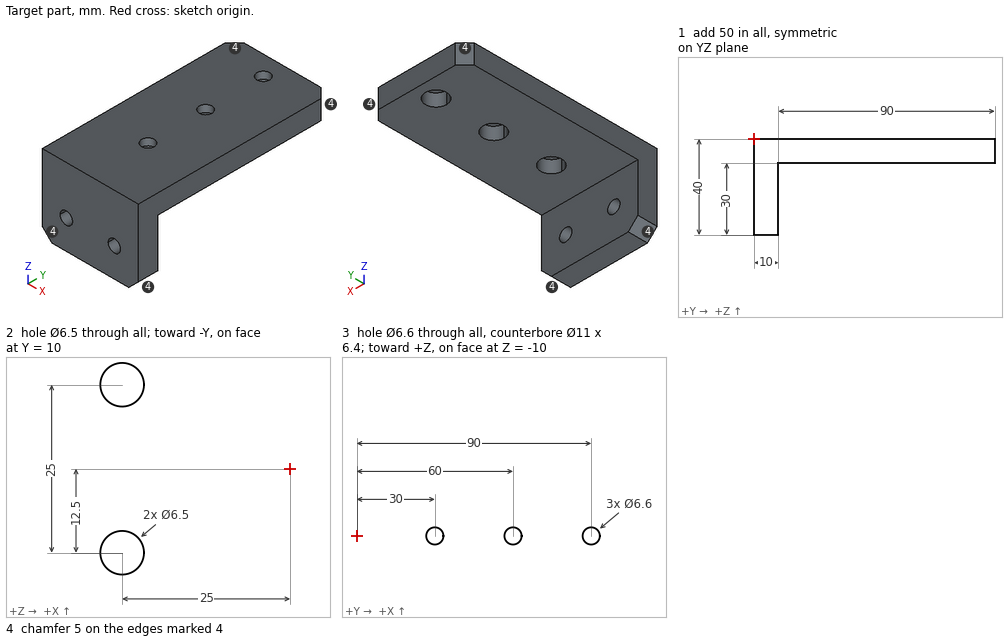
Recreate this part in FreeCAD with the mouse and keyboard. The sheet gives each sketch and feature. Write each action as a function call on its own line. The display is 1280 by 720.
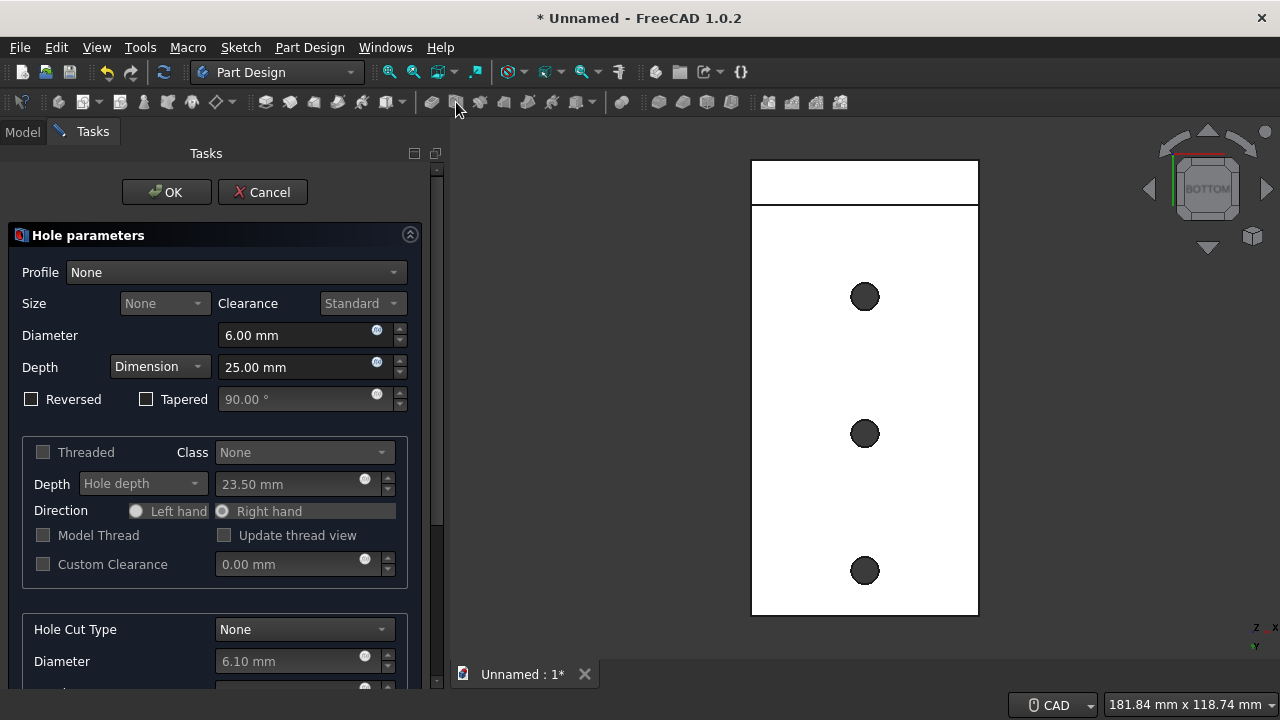
triple_click(305, 335)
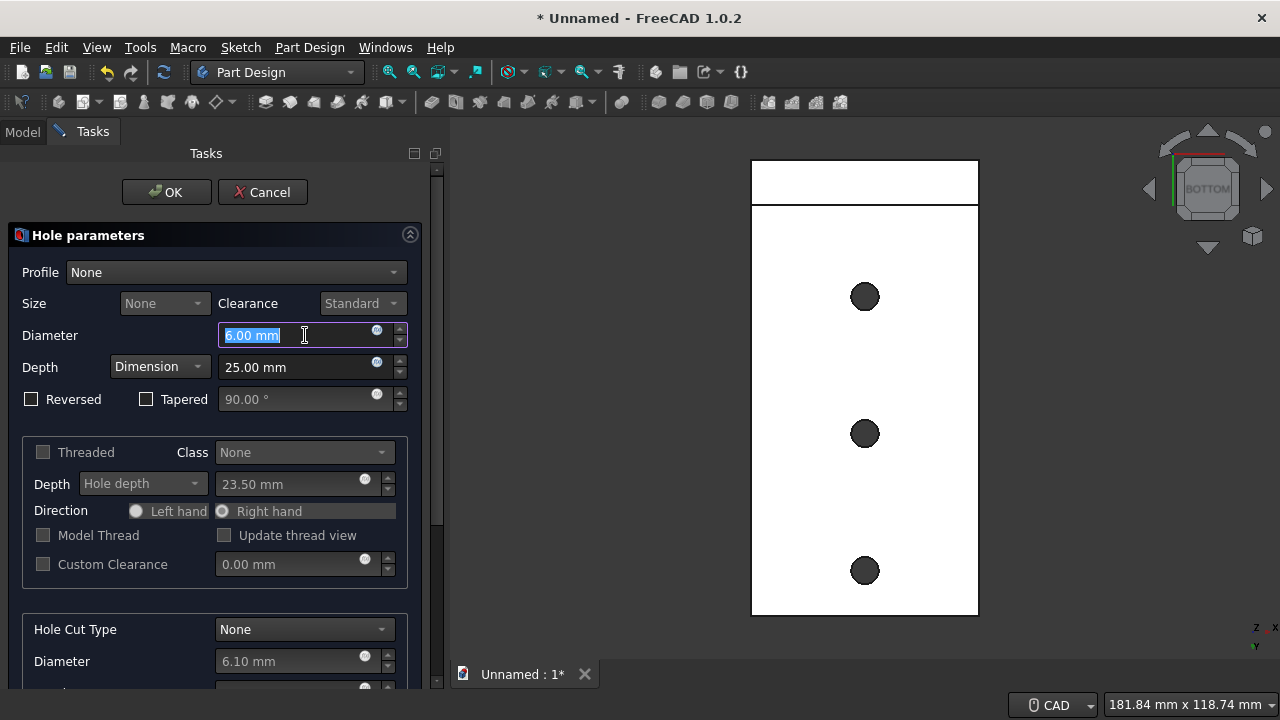
text(6.6)
key(Tab)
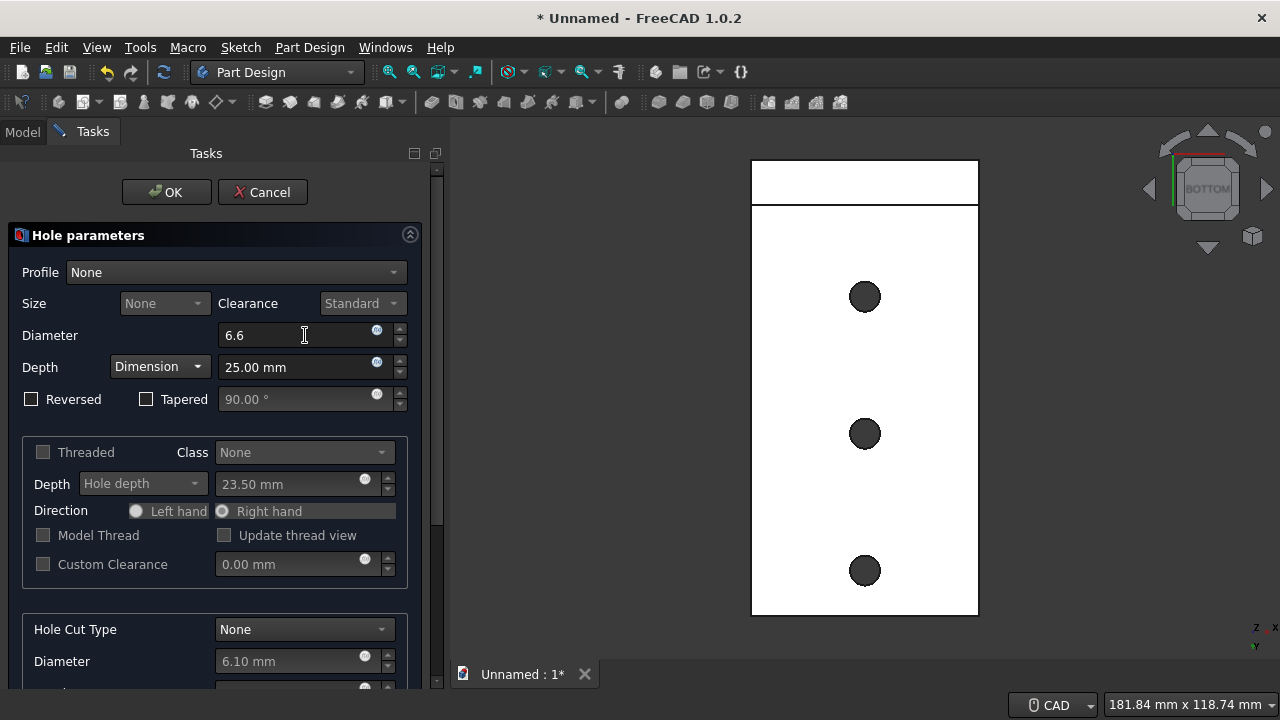
click(161, 366)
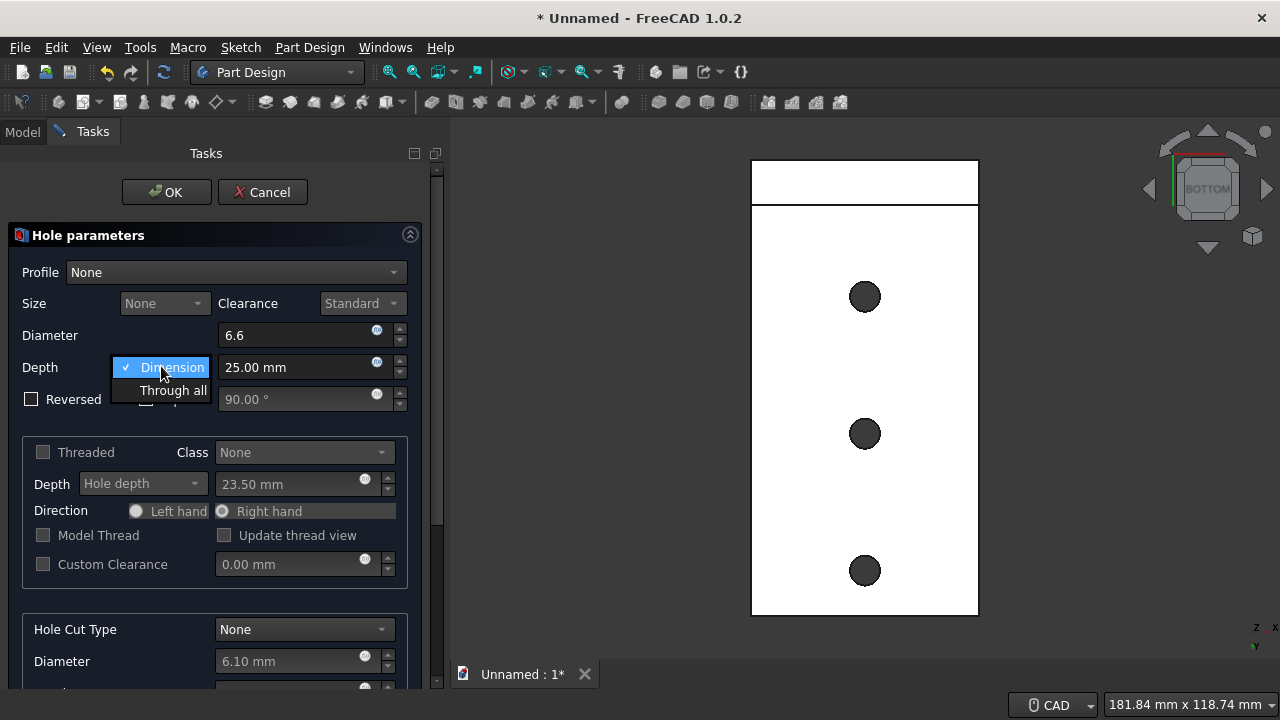
click(160, 390)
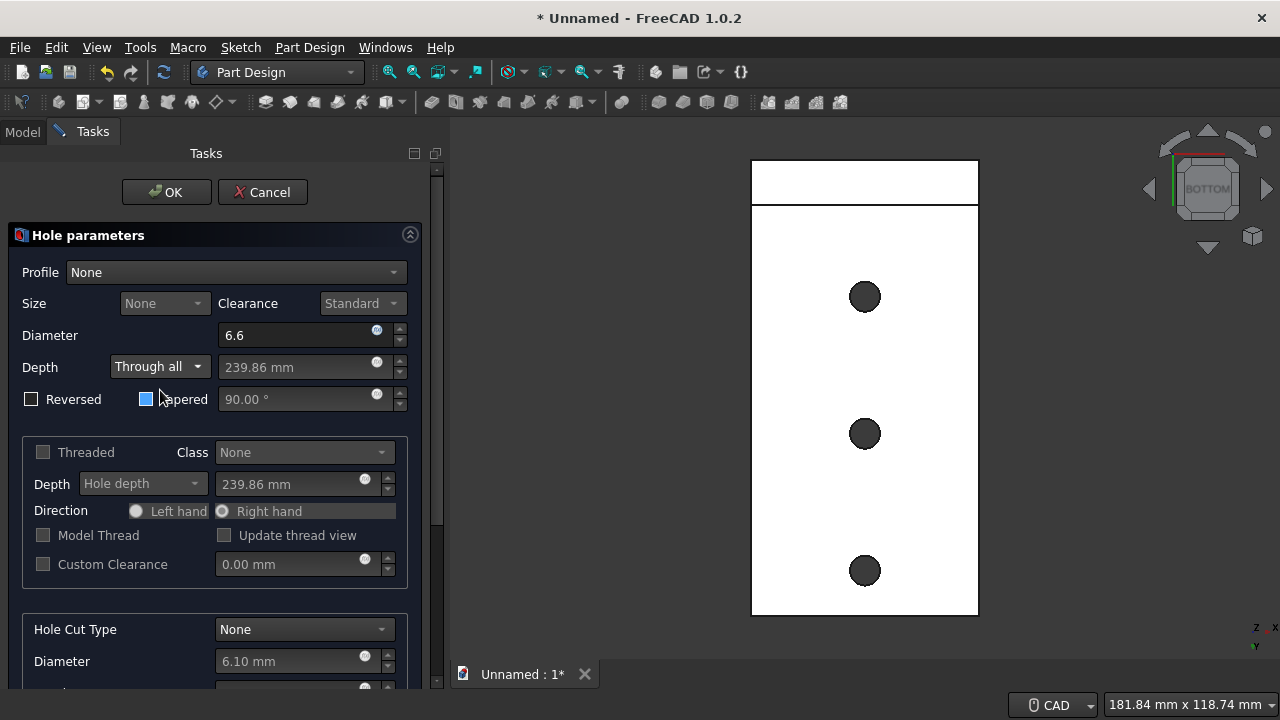
click(306, 630)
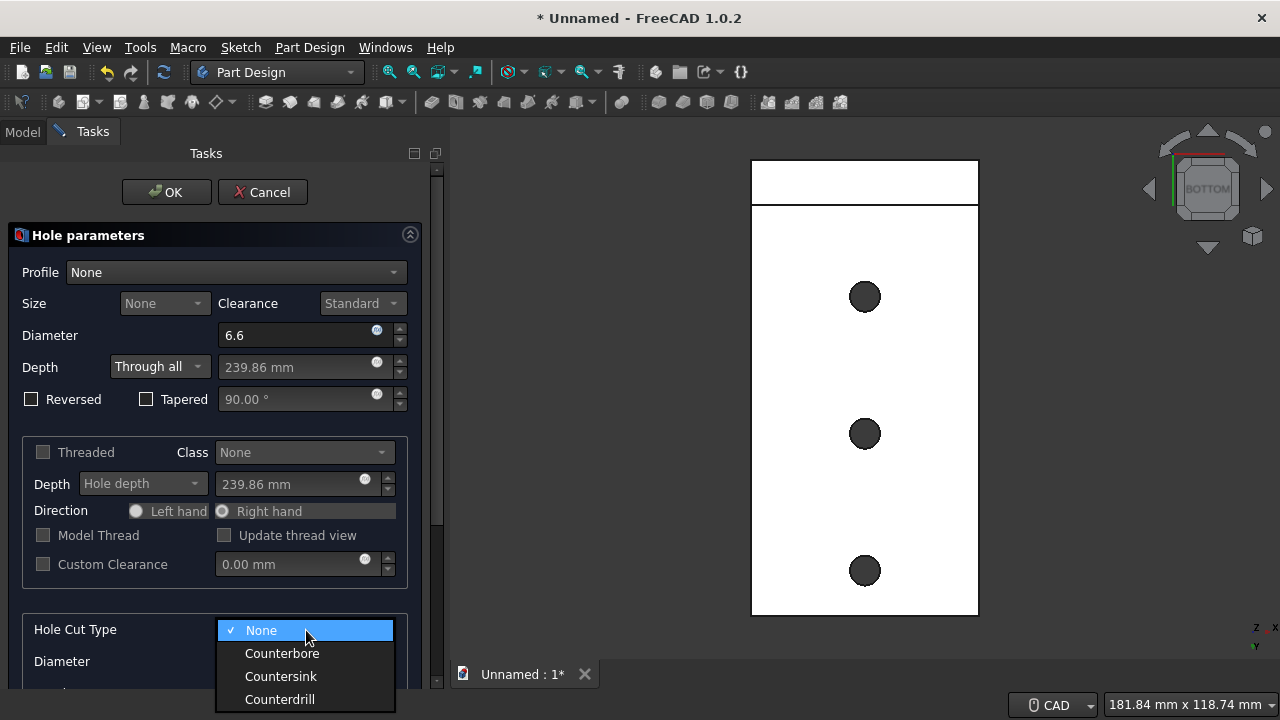
click(304, 654)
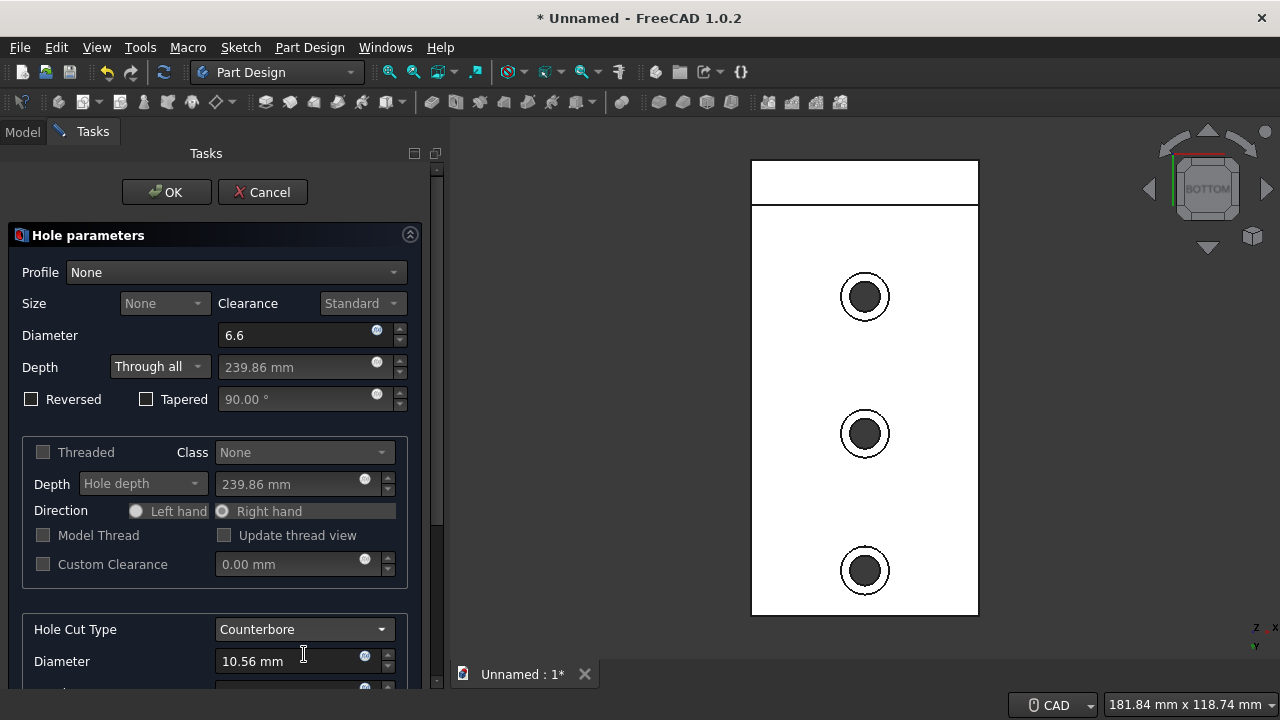
triple_click(298, 661)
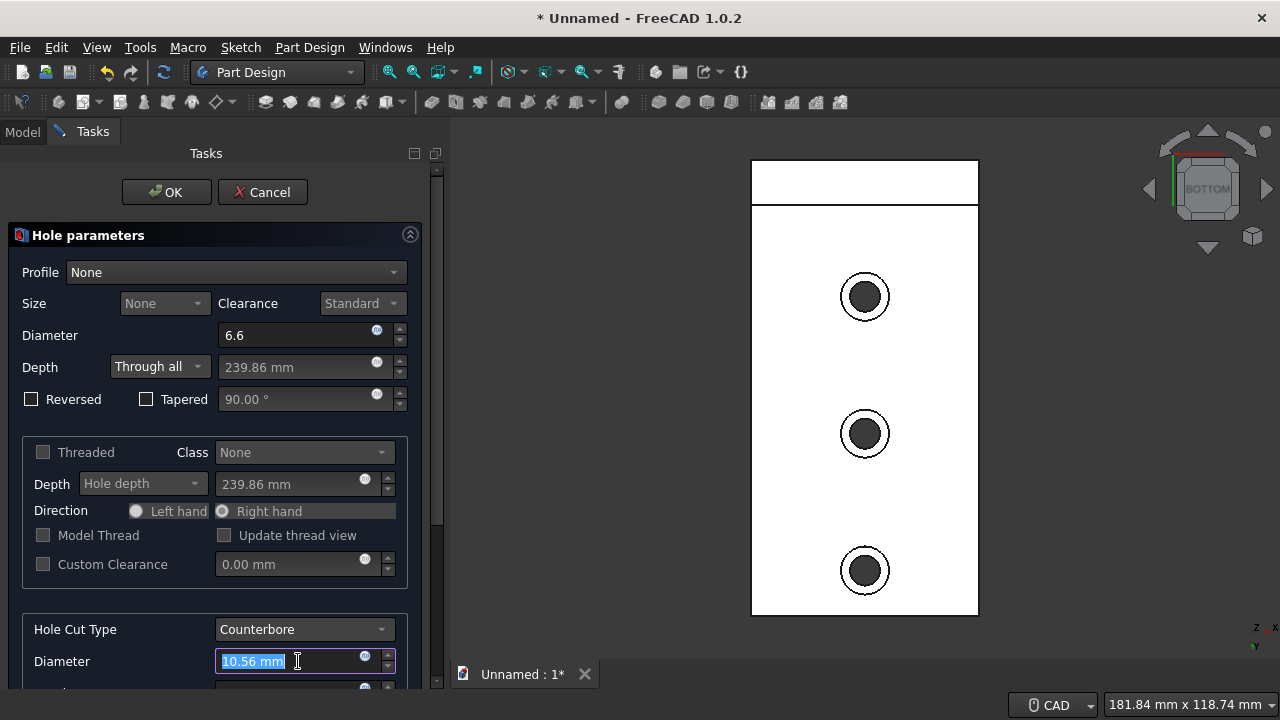
text(11)
key(Tab)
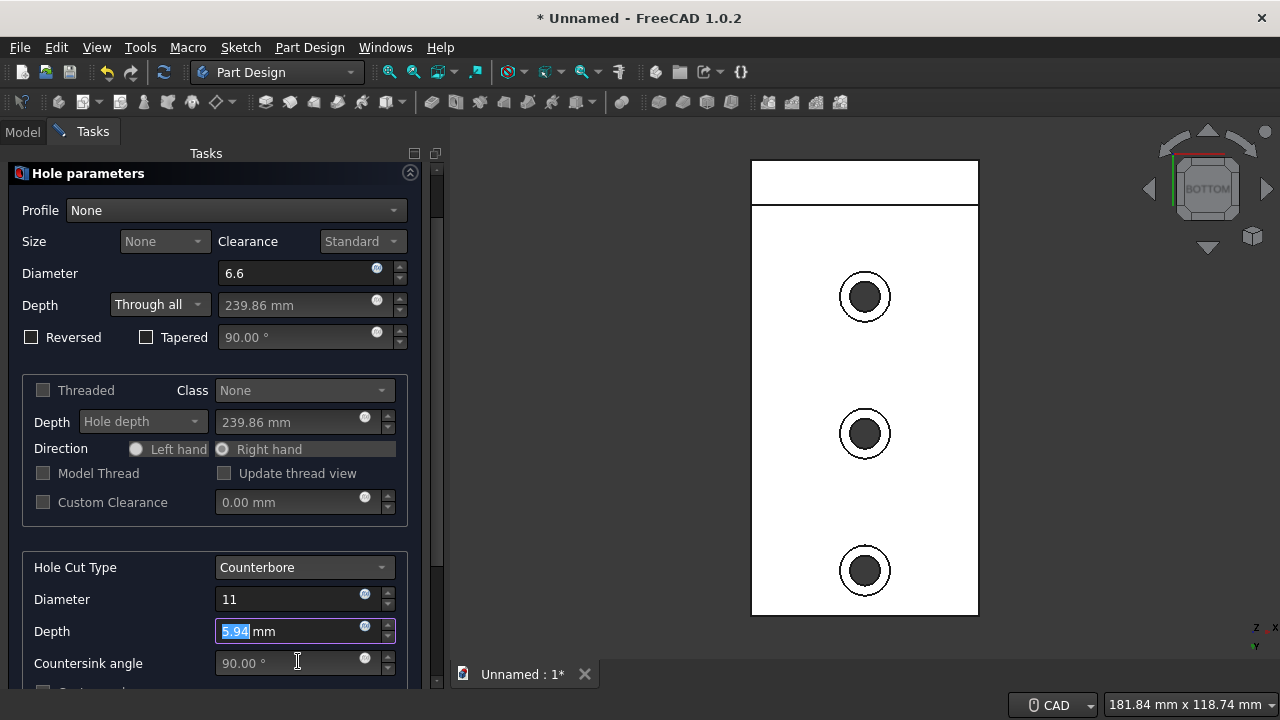
text(6.4)
key(Tab)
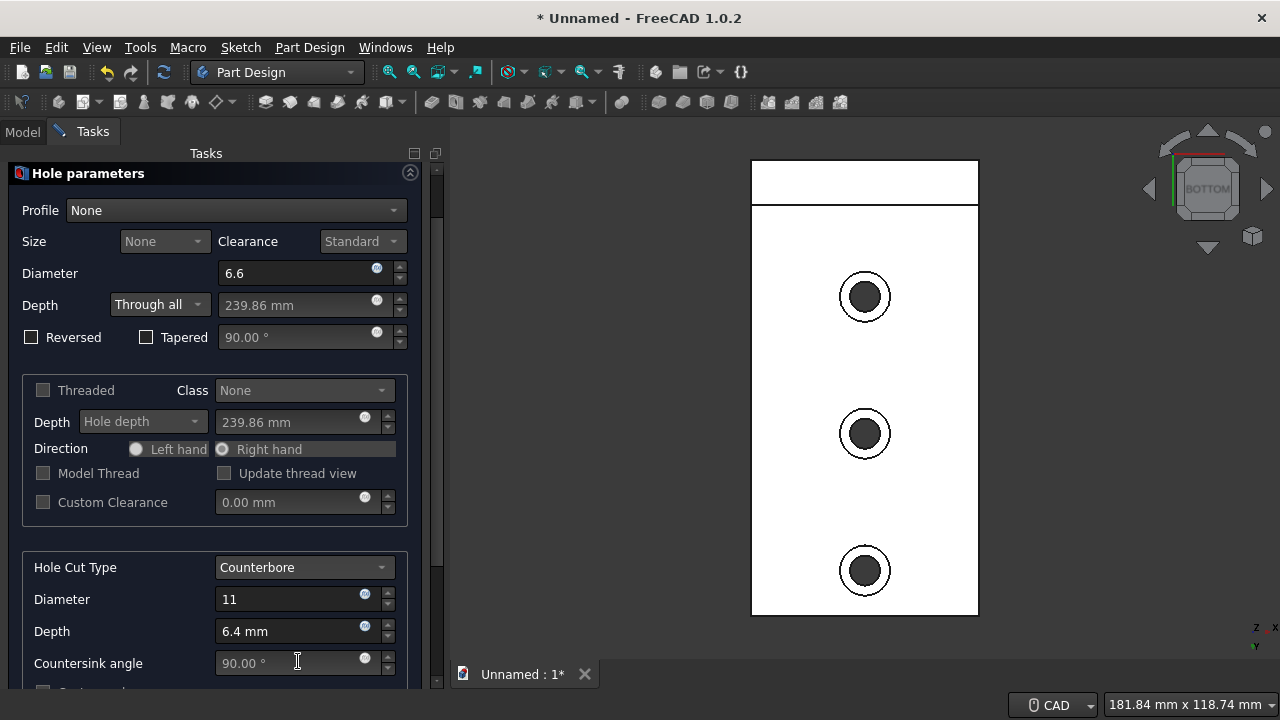
scroll(437, 426, up, 2)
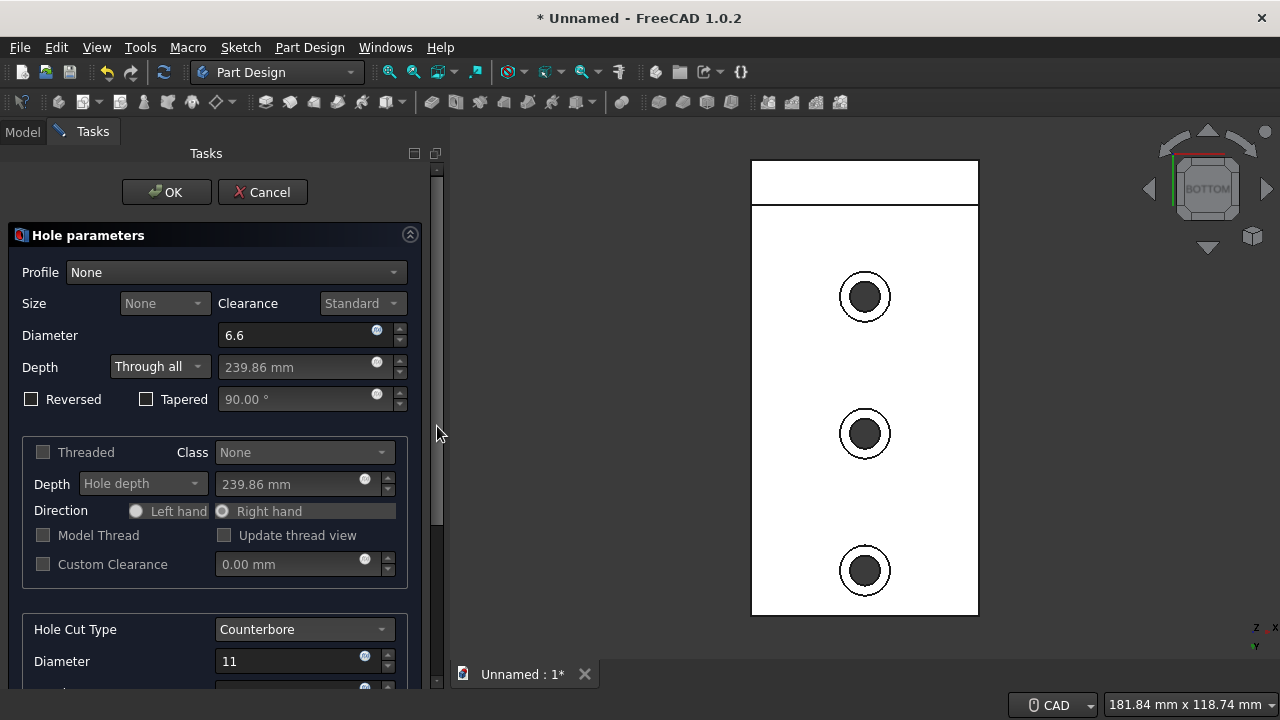
click(167, 192)